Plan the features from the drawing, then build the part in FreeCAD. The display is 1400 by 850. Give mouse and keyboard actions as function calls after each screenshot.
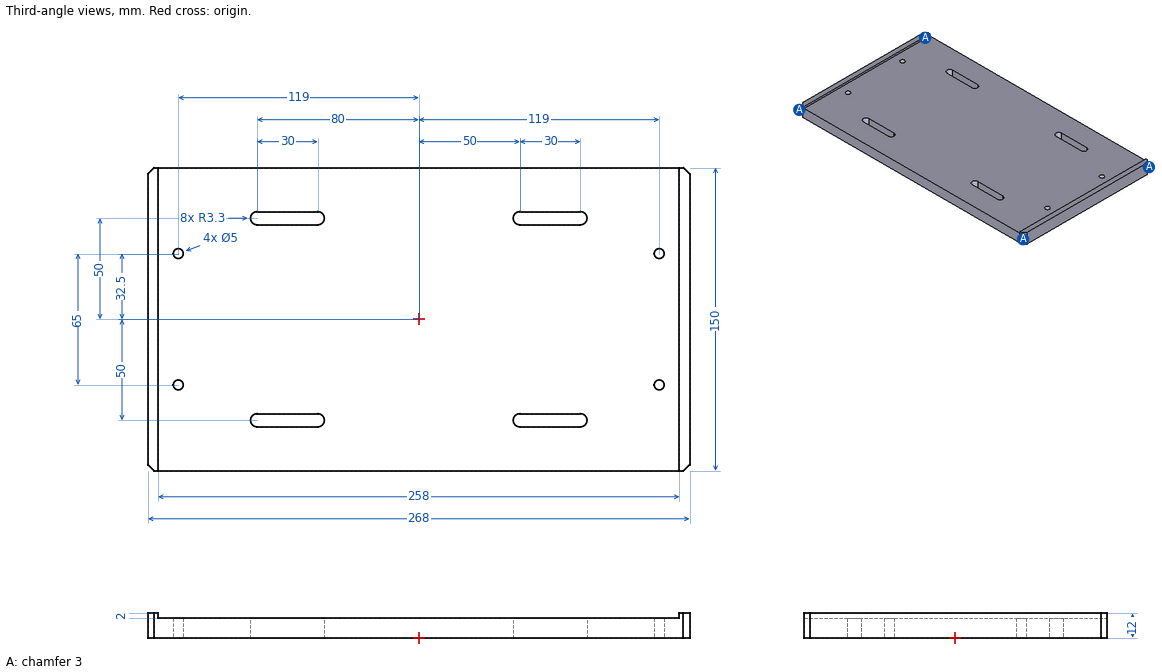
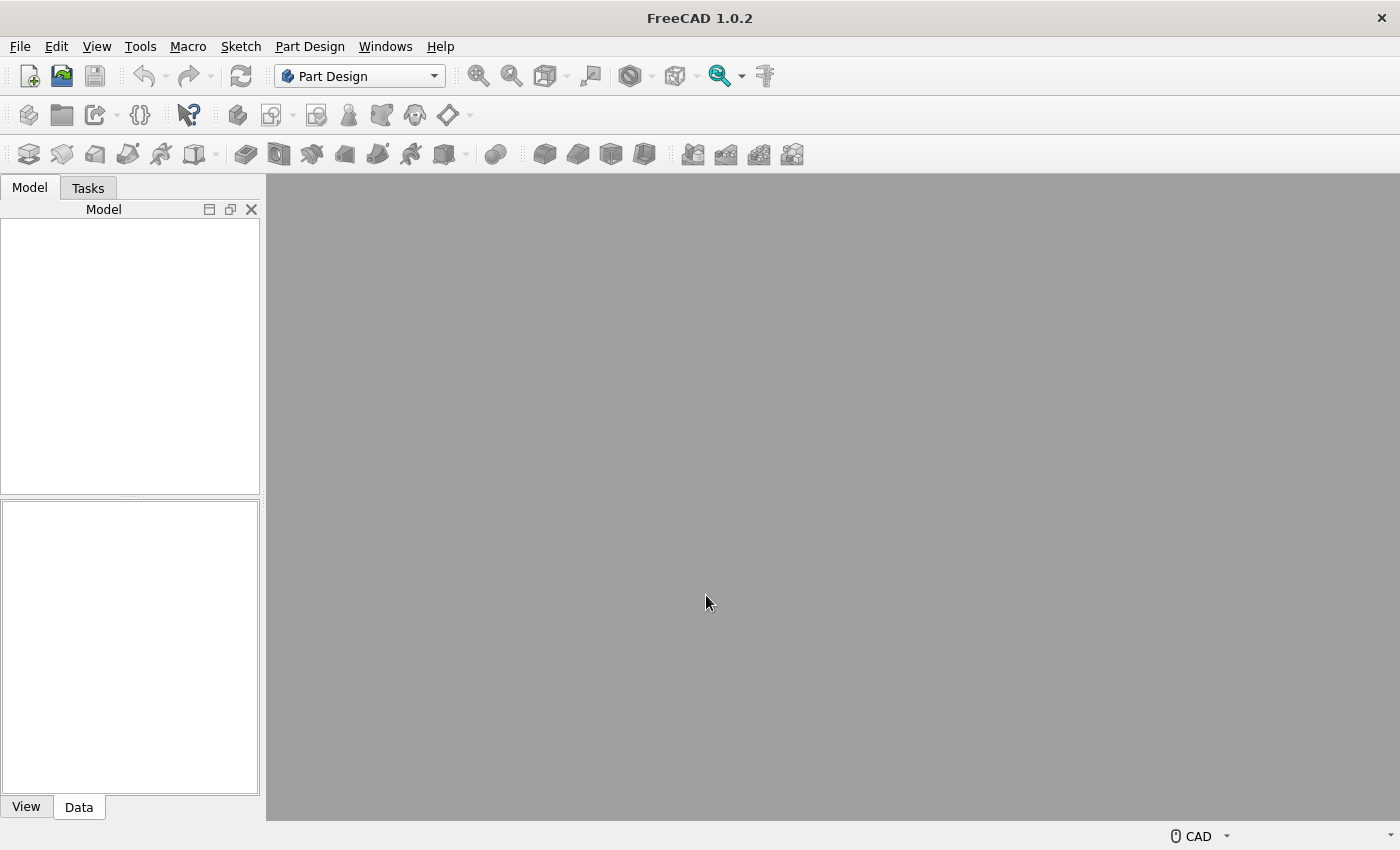
click(29, 76)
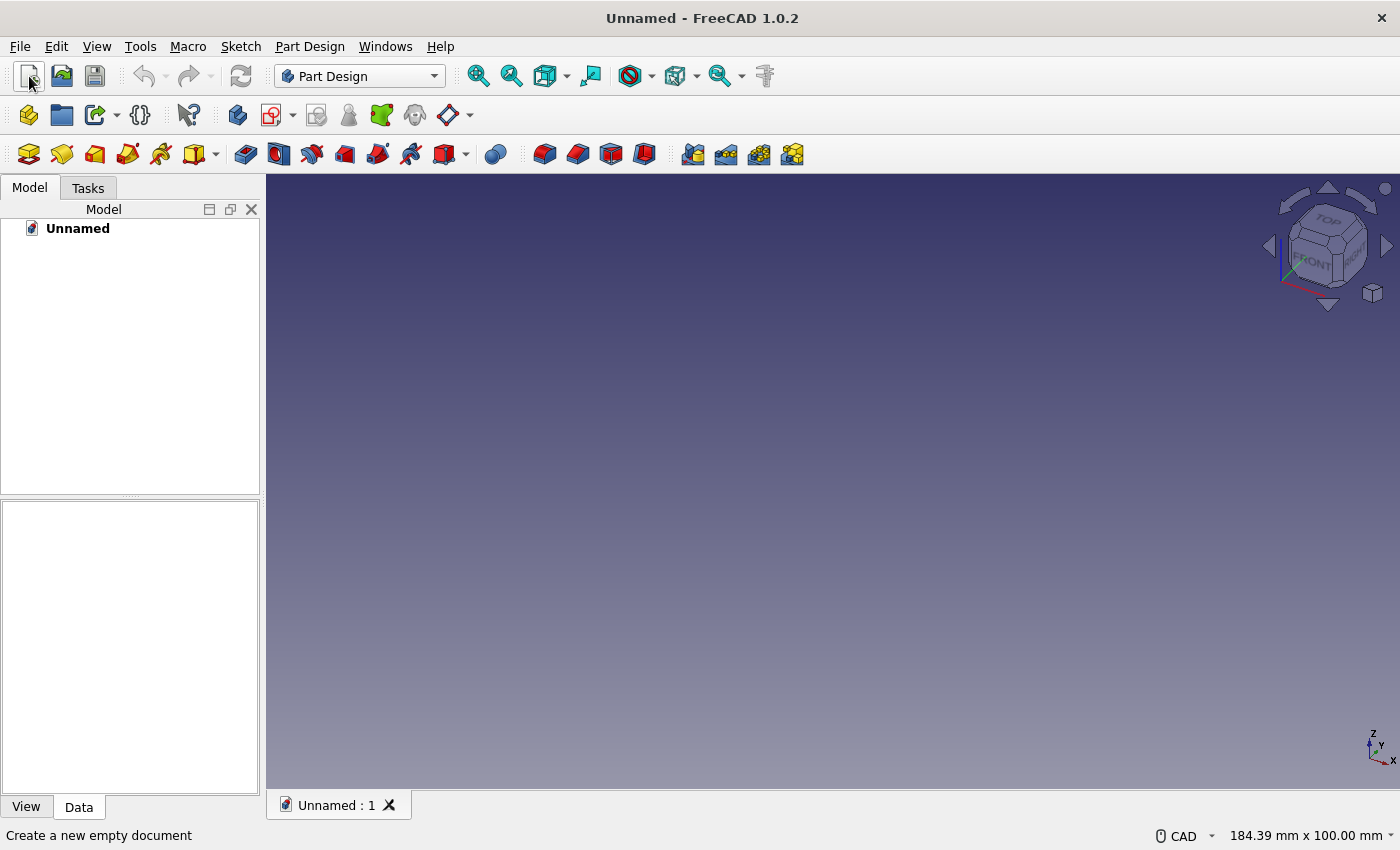
click(270, 116)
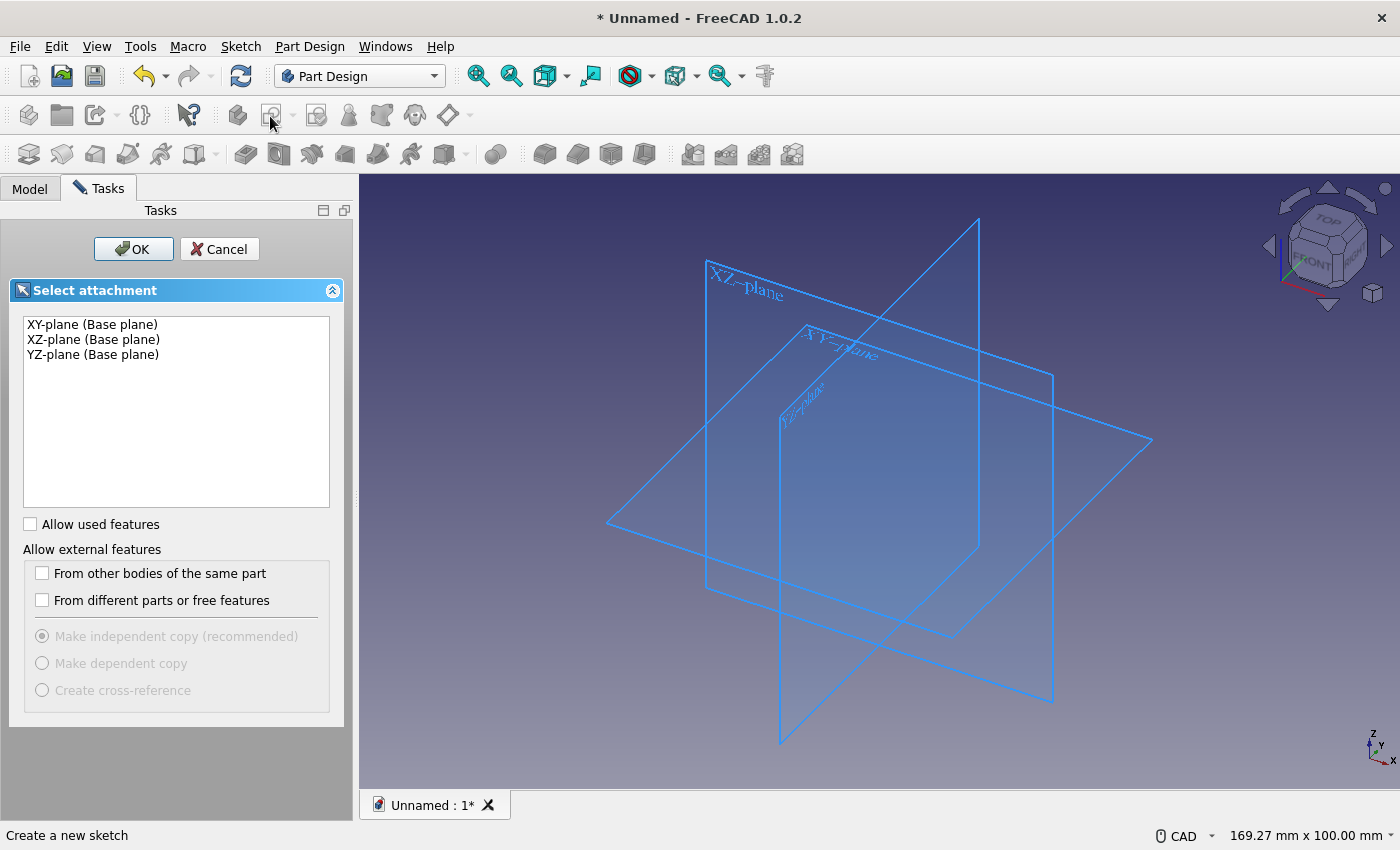
click(84, 324)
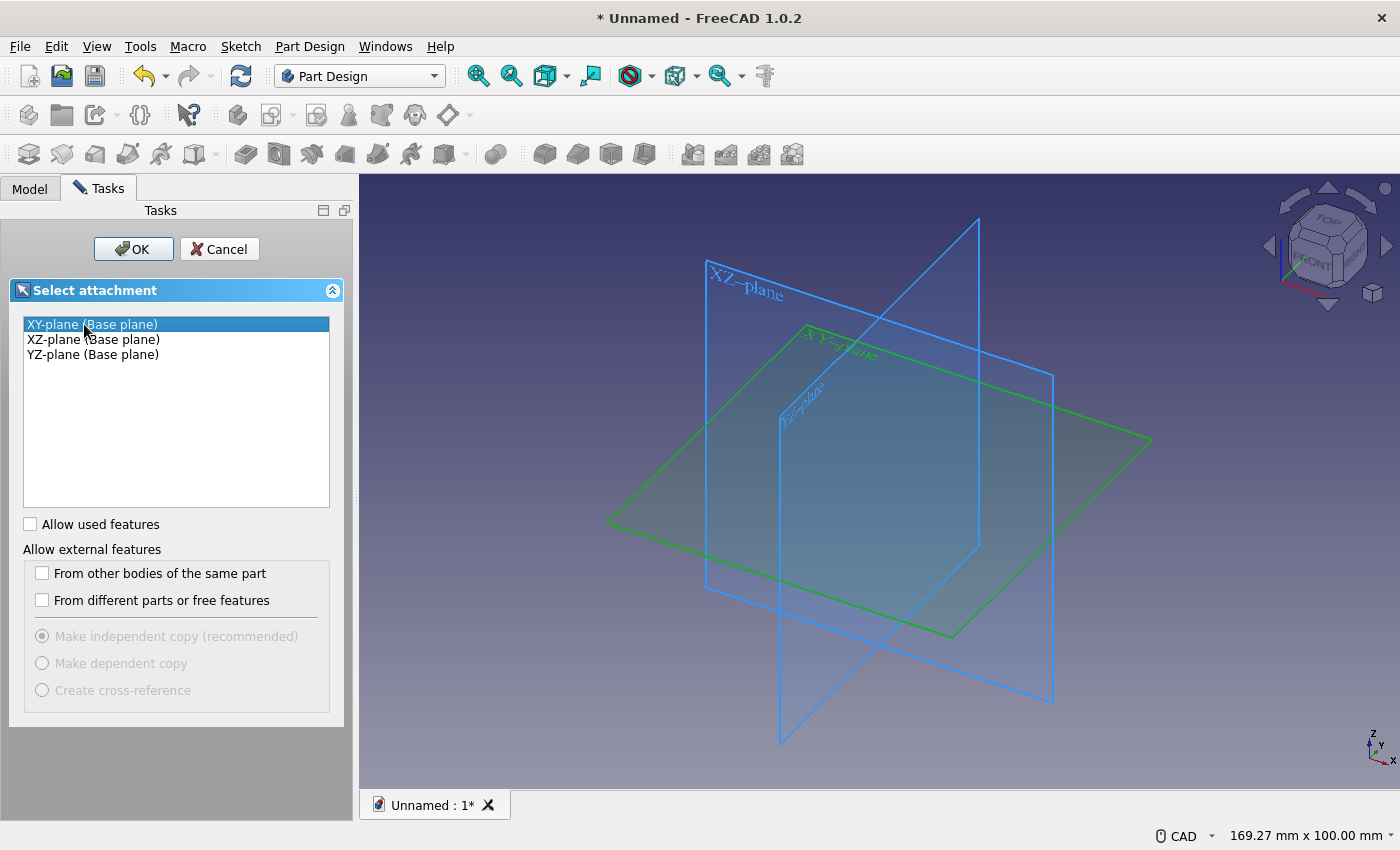
click(134, 249)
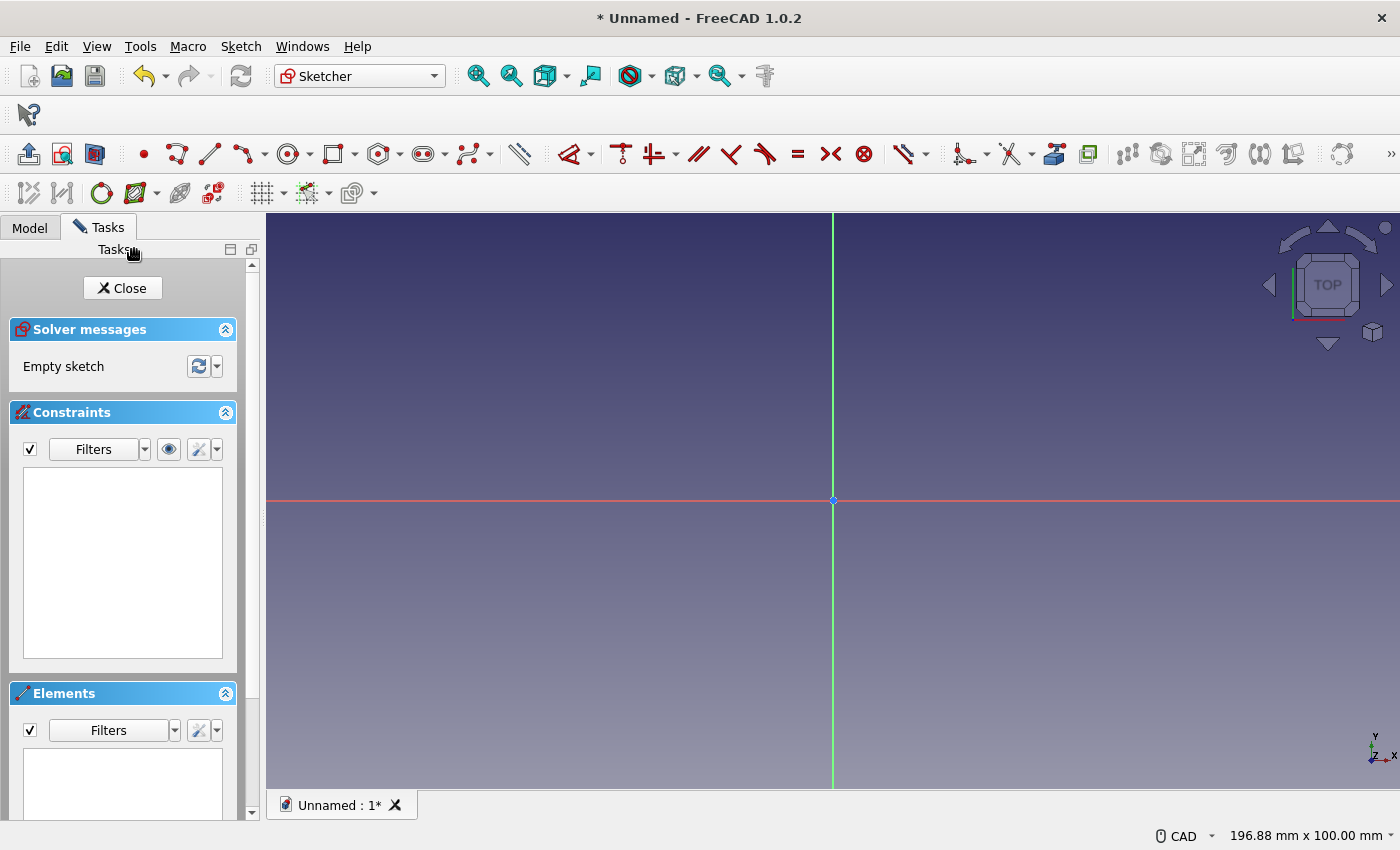
scroll(709, 501, down, 4)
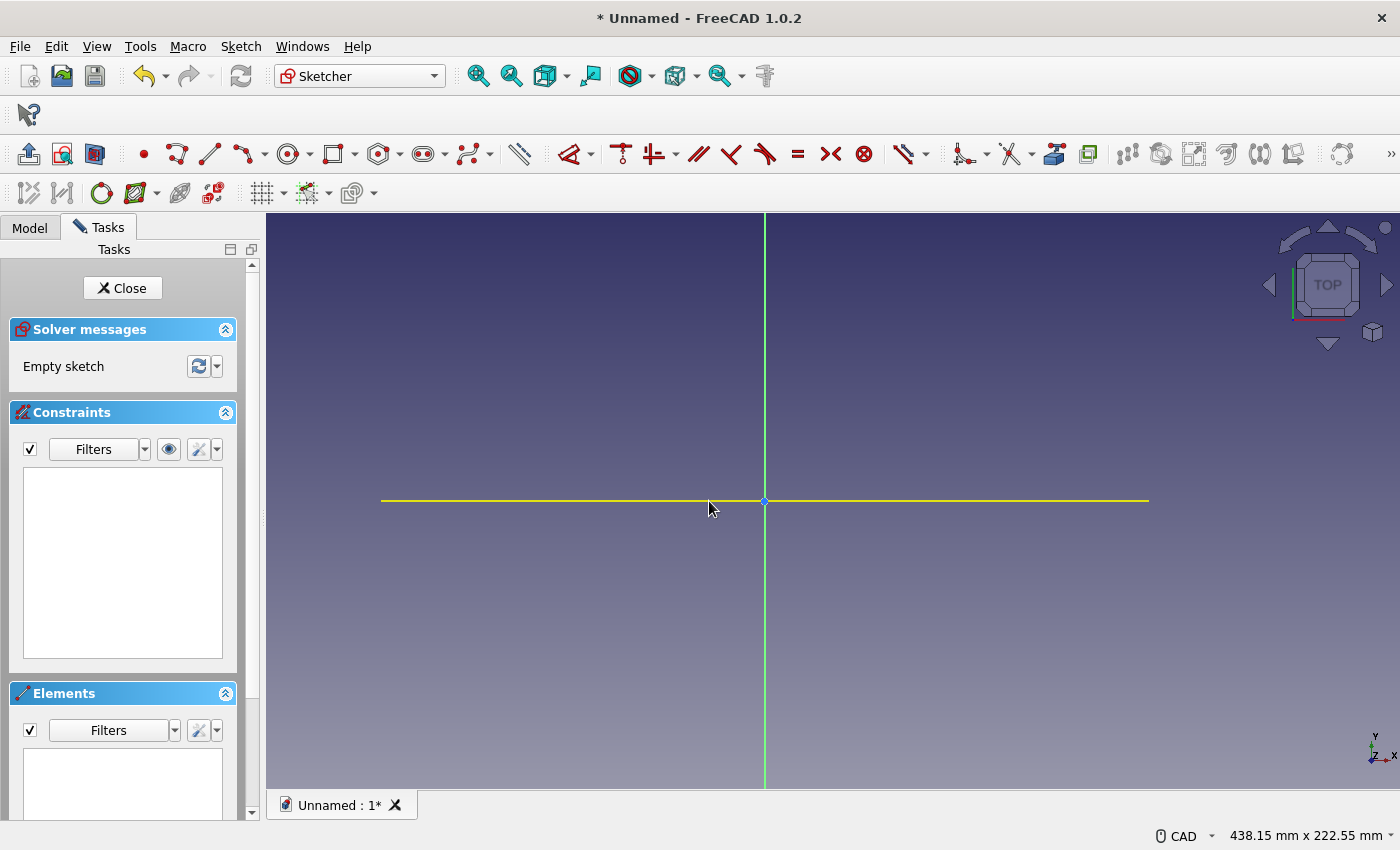
key(g)
key(v)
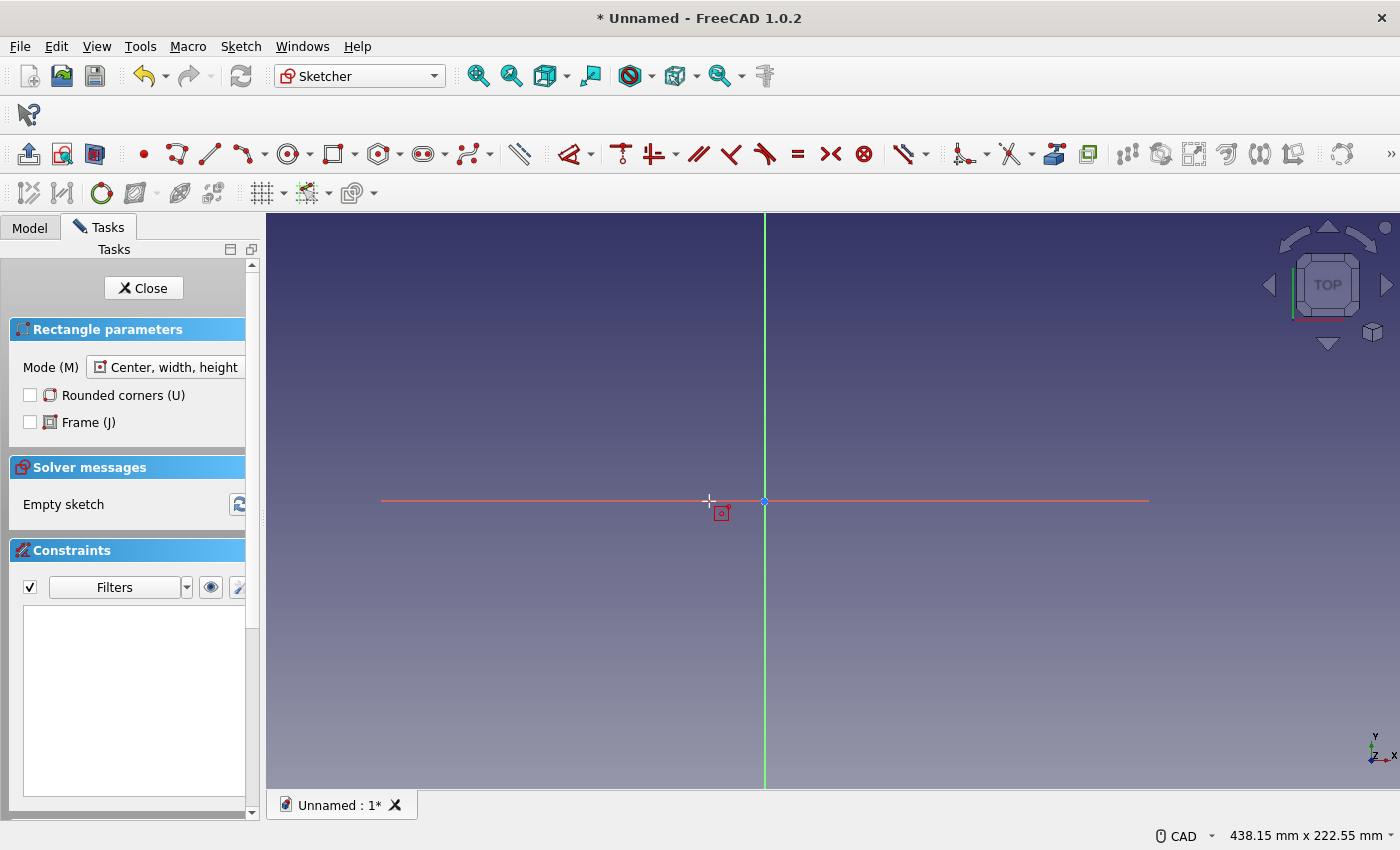
click(765, 501)
move(1112, 307)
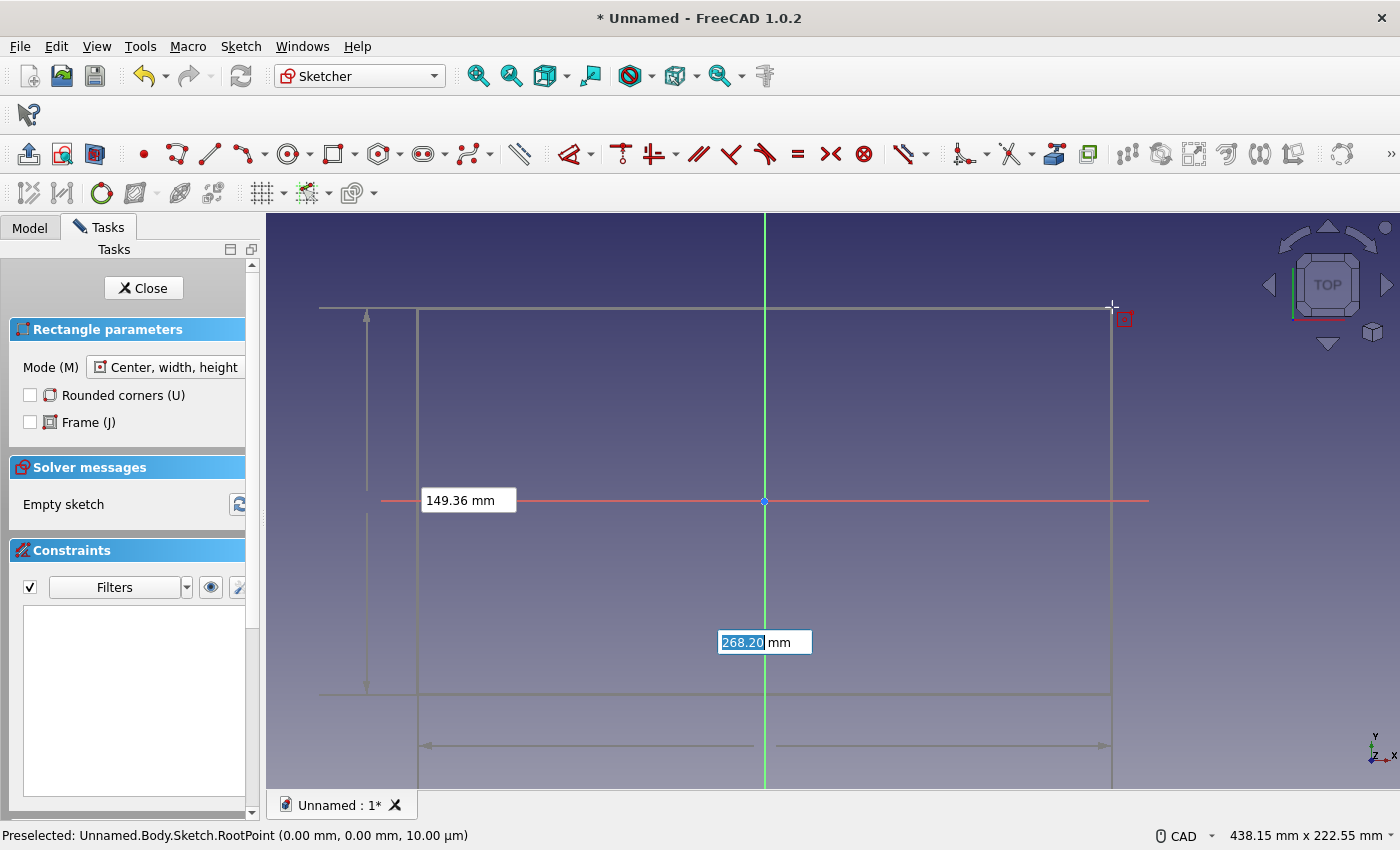
text(268)
key(Tab)
text(150)
key(Return)
key(Escape)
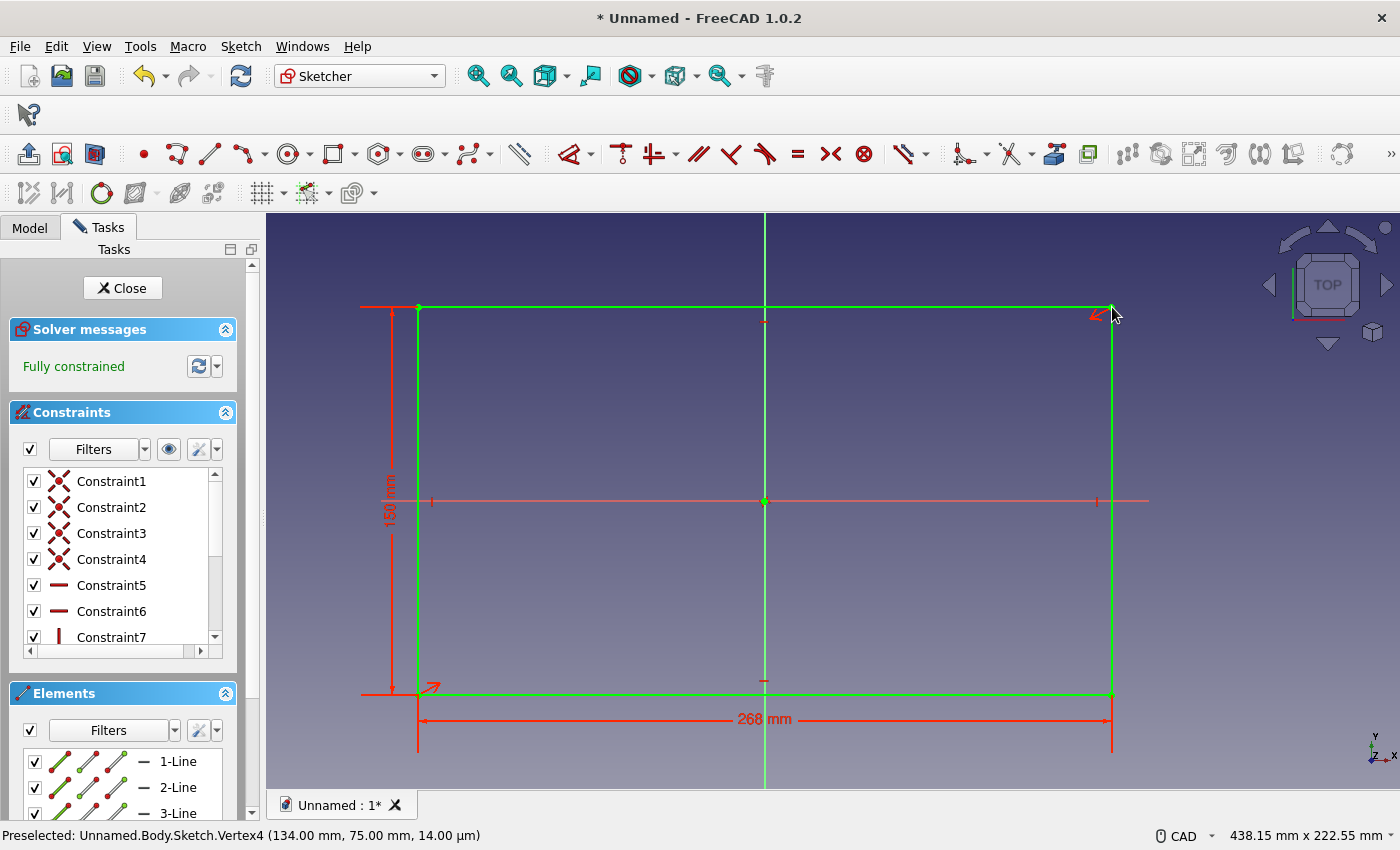
click(123, 288)